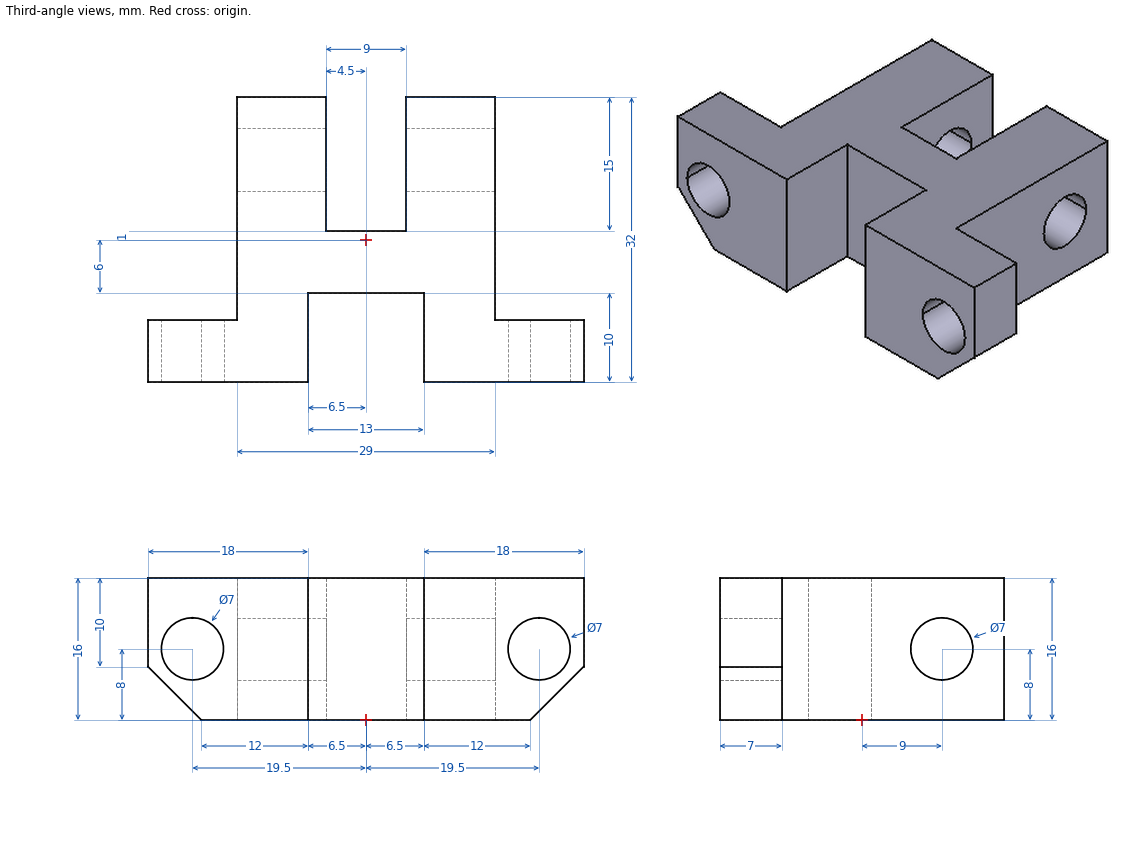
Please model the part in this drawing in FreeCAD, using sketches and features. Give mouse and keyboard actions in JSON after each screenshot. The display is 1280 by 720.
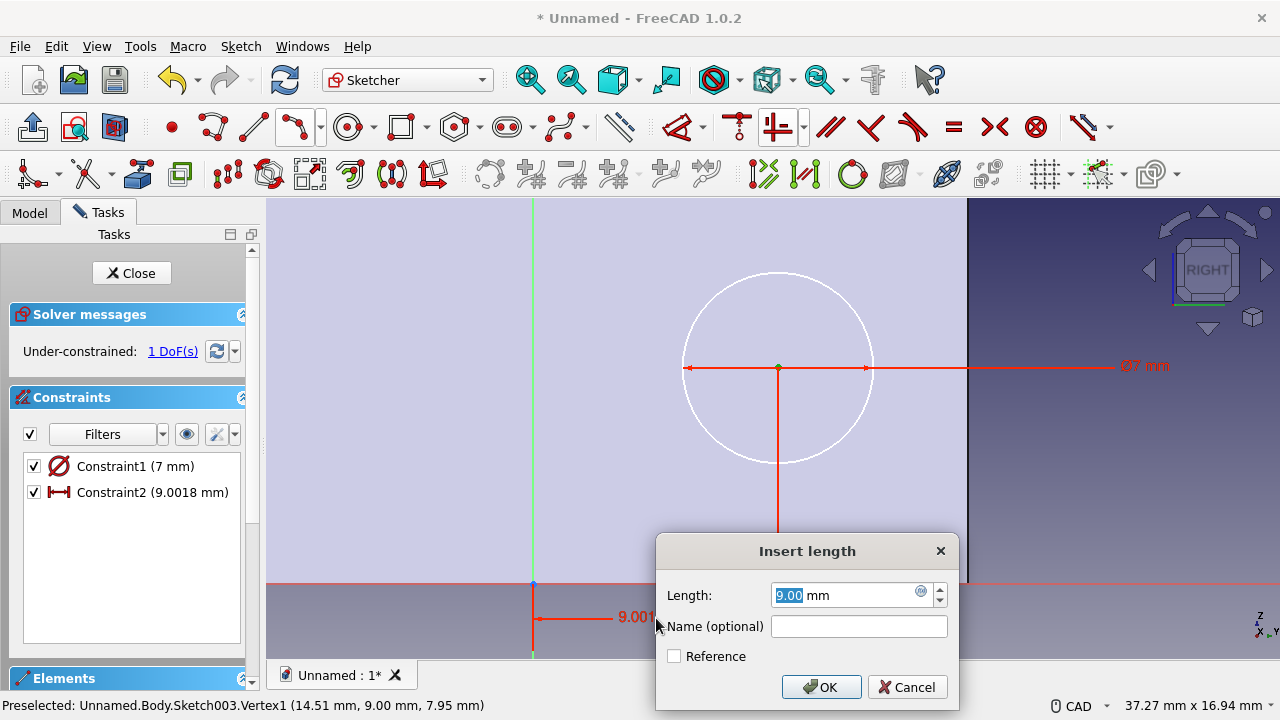
{"action": "type", "text": "9"}
{"action": "key", "text": "Return"}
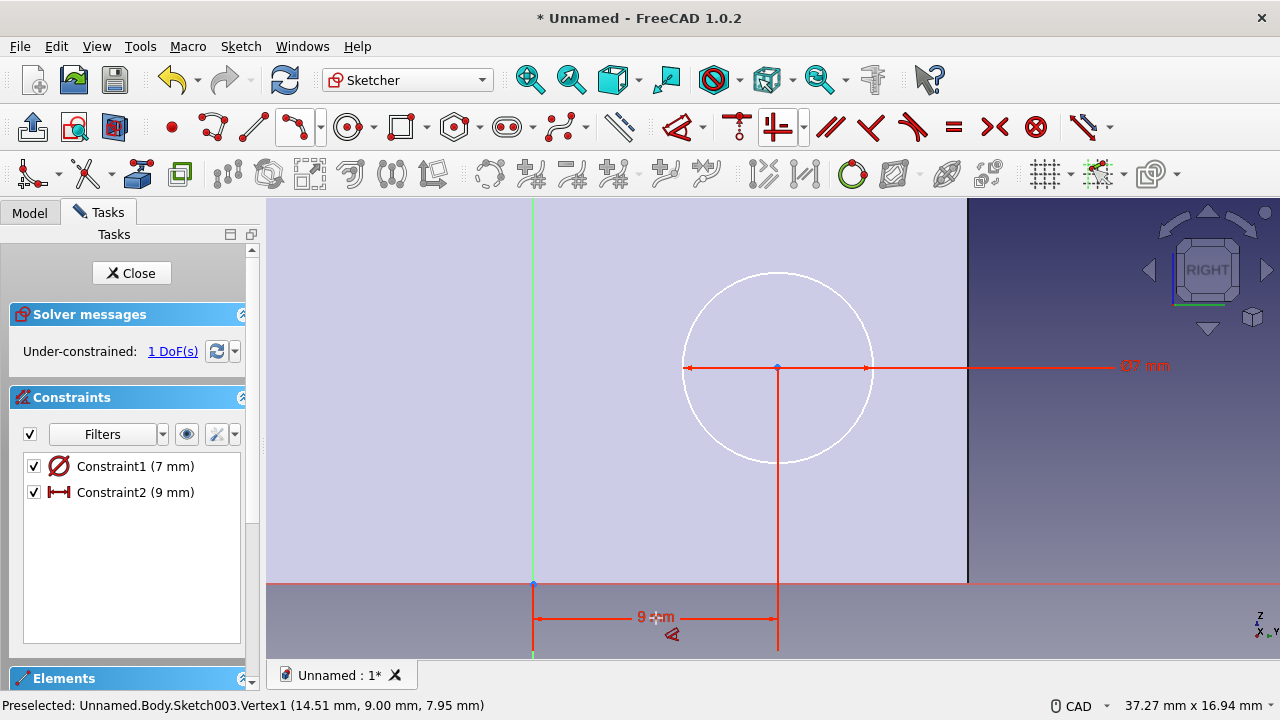
{"action": "left_click", "coordinate": [778, 368]}
{"action": "left_click", "coordinate": [499, 476]}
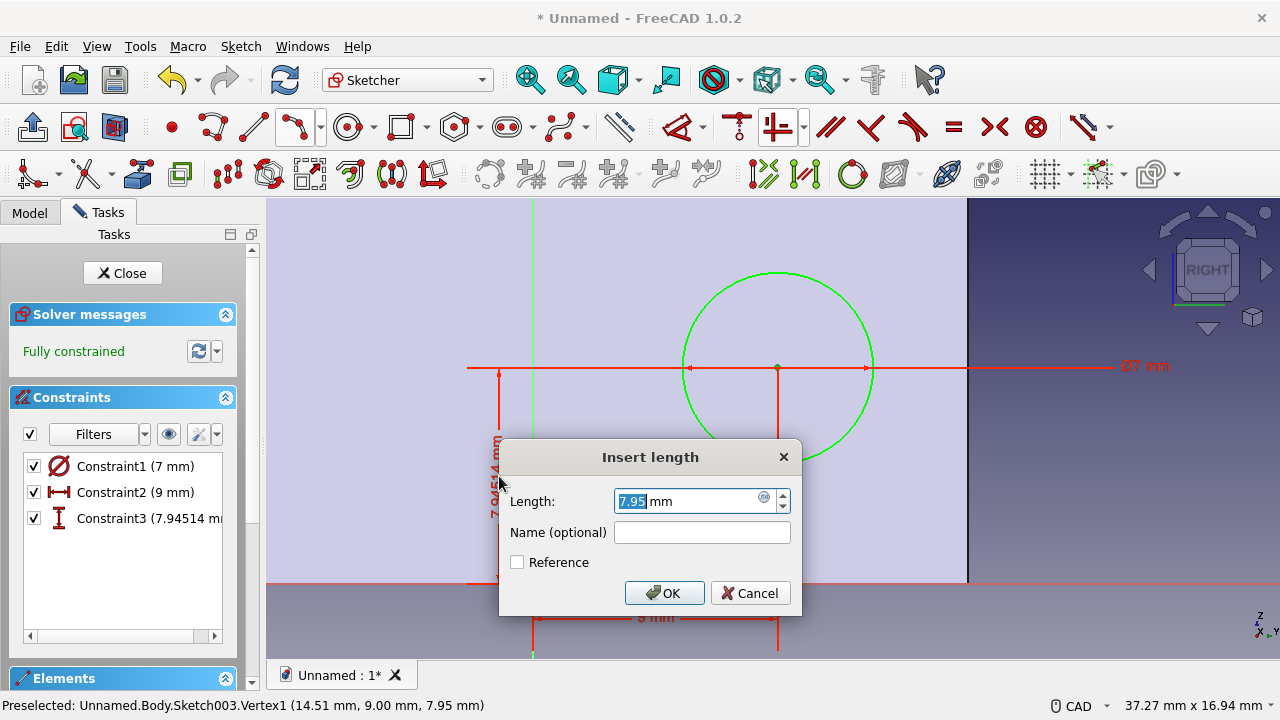
{"action": "type", "text": "8"}
{"action": "key", "text": "Return"}
{"action": "key", "text": "Escape"}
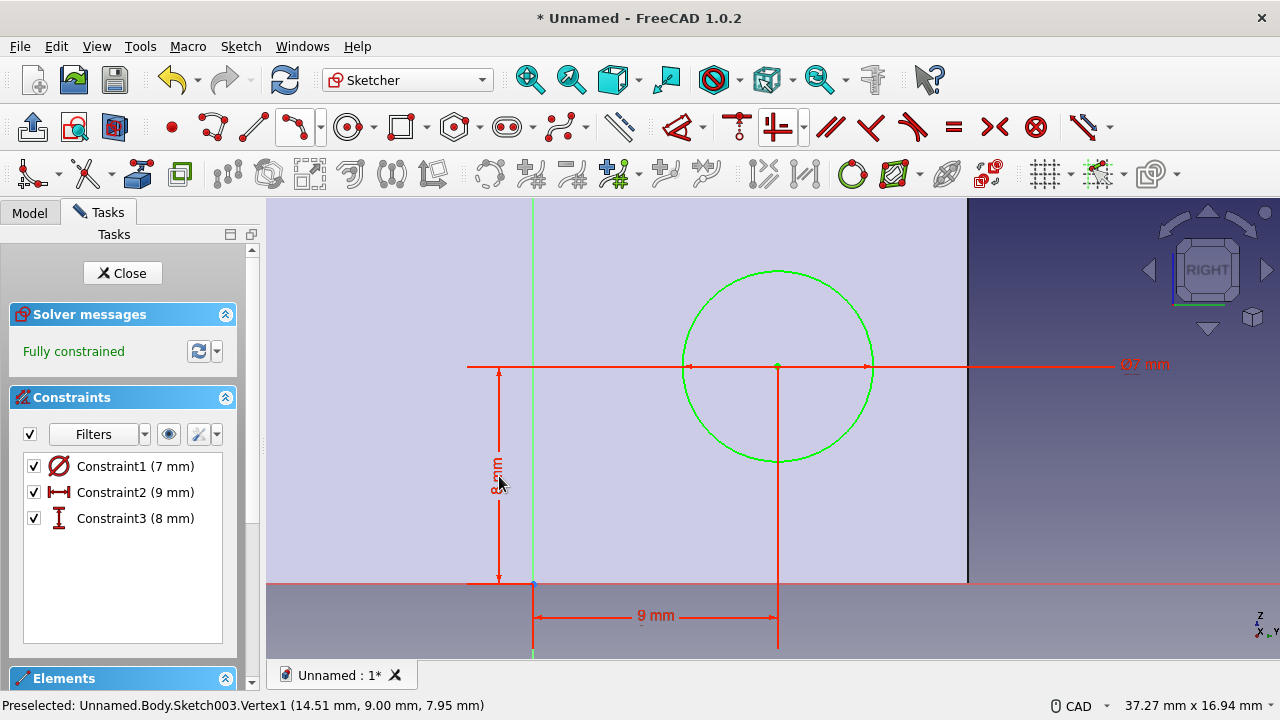
{"action": "left_click", "coordinate": [123, 273]}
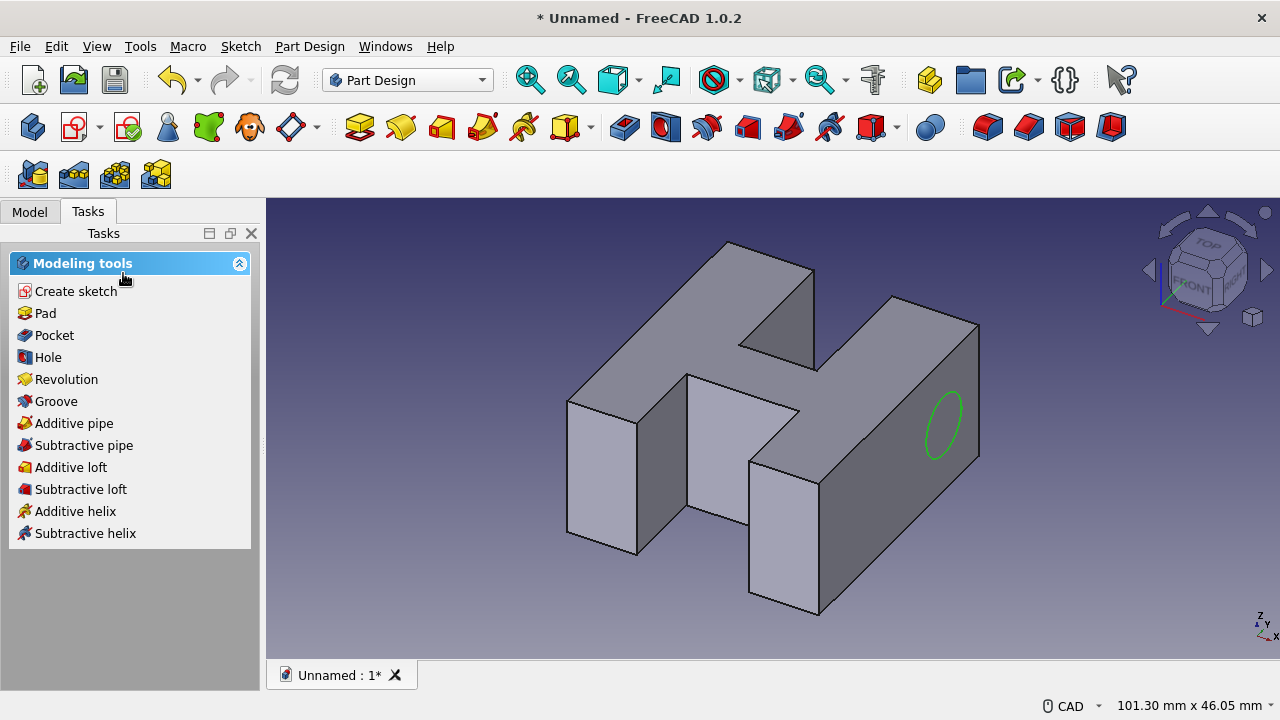
{"action": "left_click", "coordinate": [625, 128]}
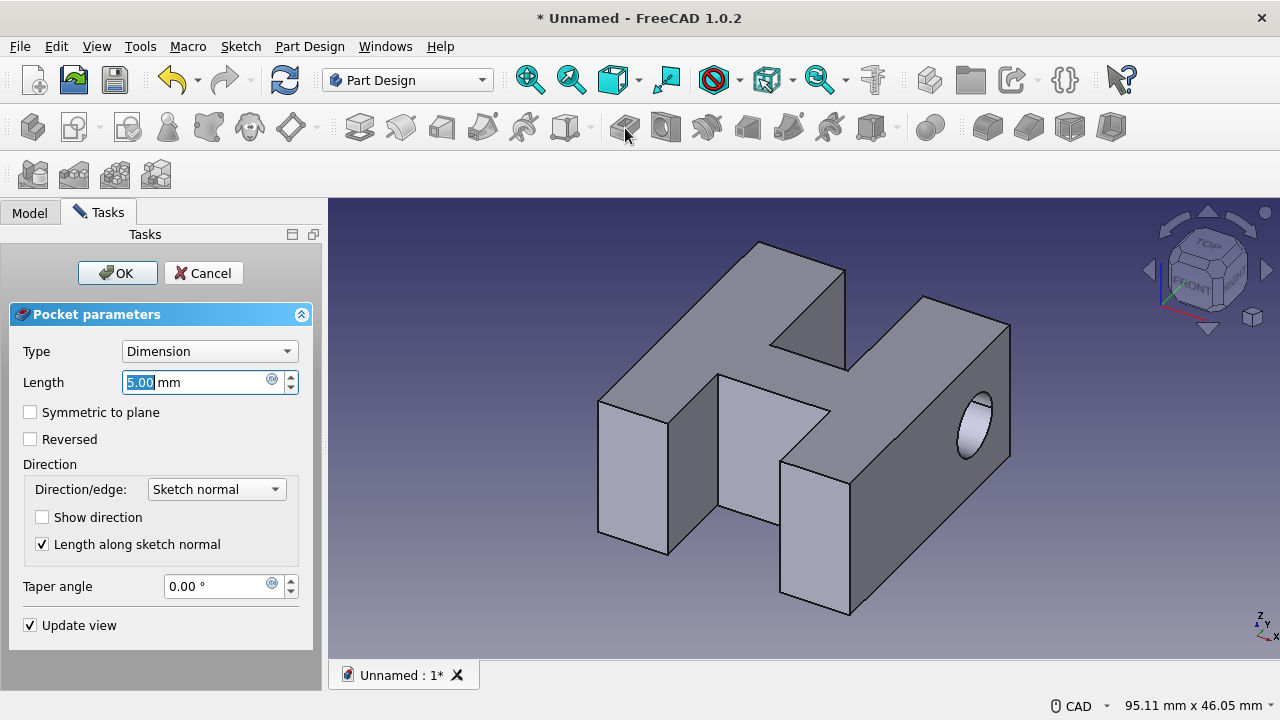
{"action": "left_click", "coordinate": [210, 352]}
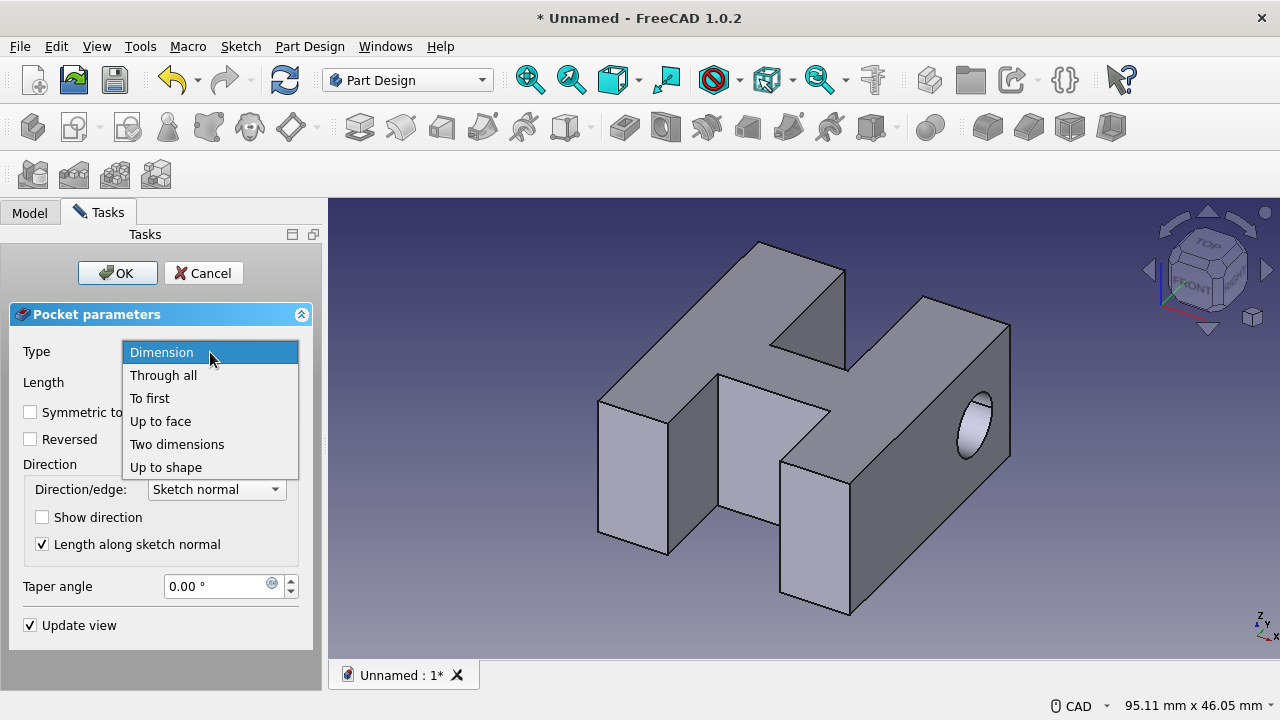
{"action": "left_click", "coordinate": [208, 376]}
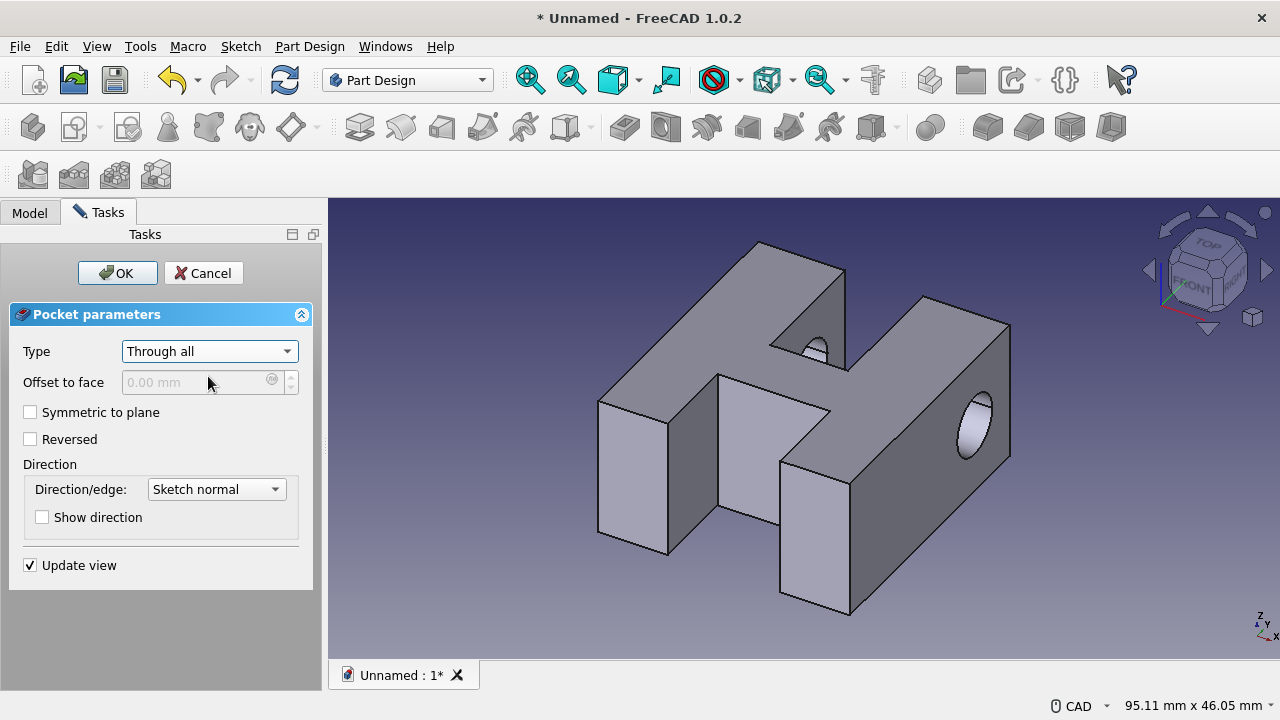
{"action": "left_click", "coordinate": [118, 273]}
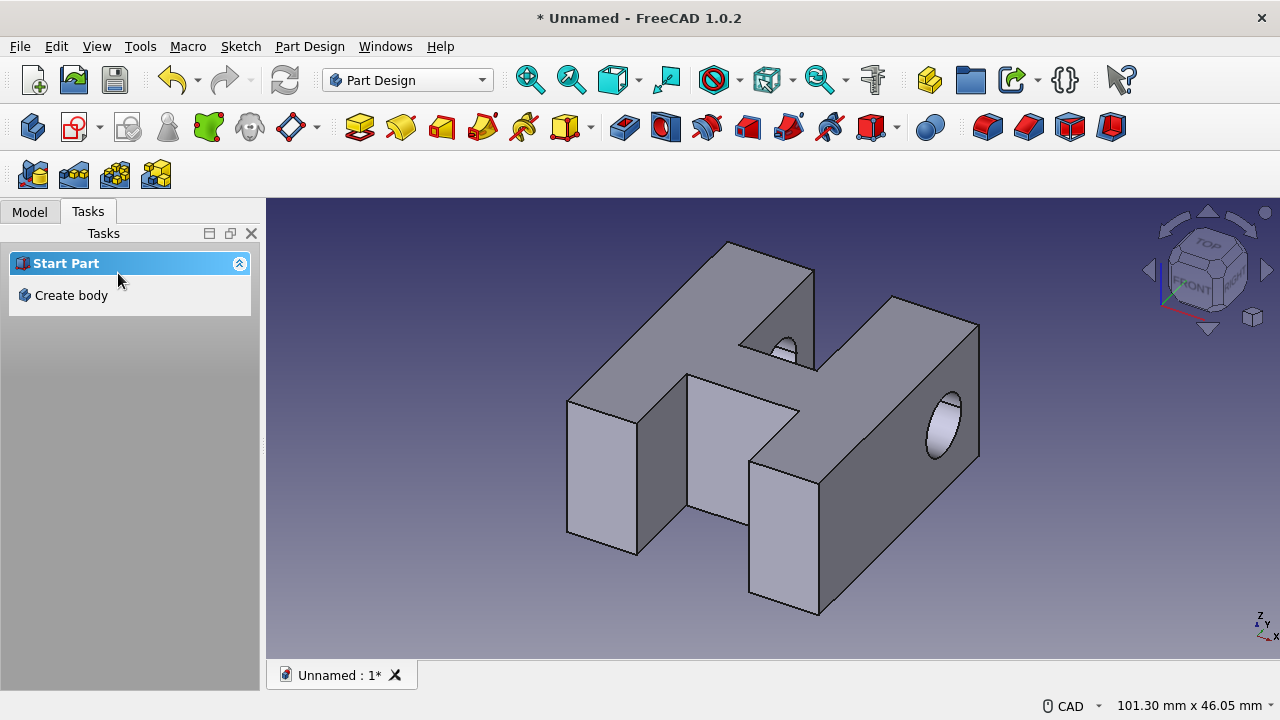
{"action": "left_click", "coordinate": [784, 518]}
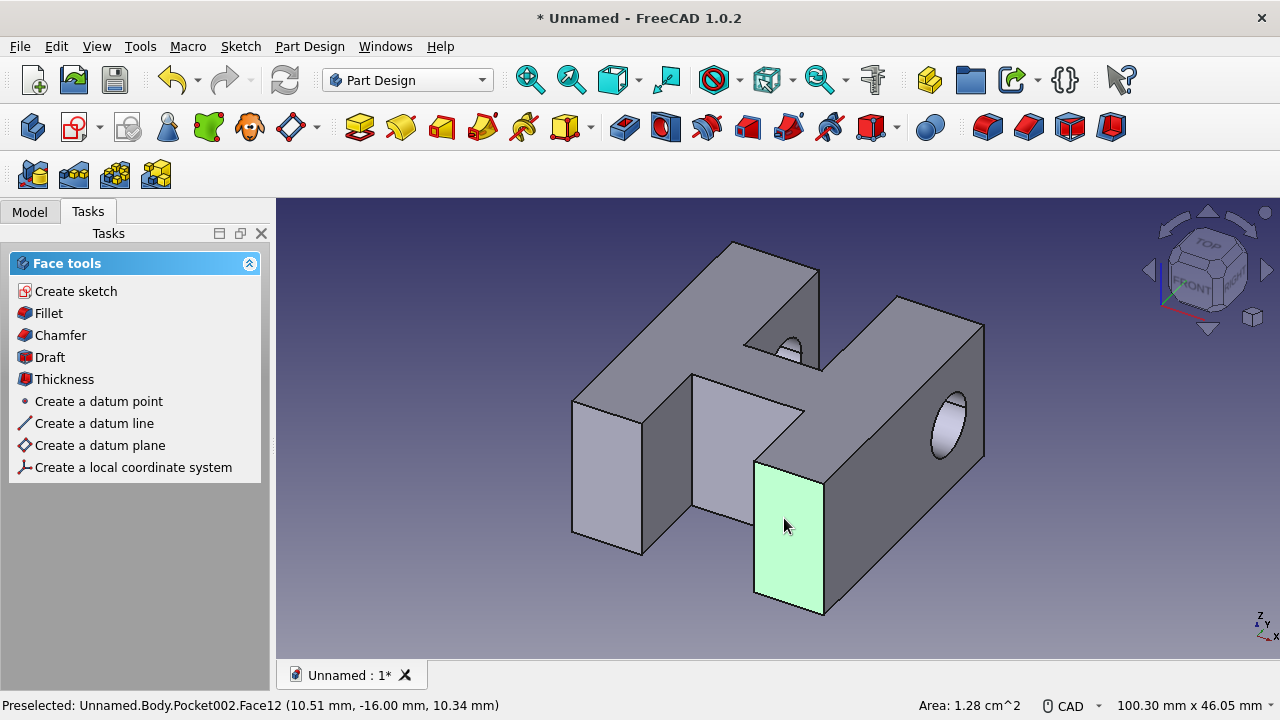
{"action": "left_click", "coordinate": [74, 128]}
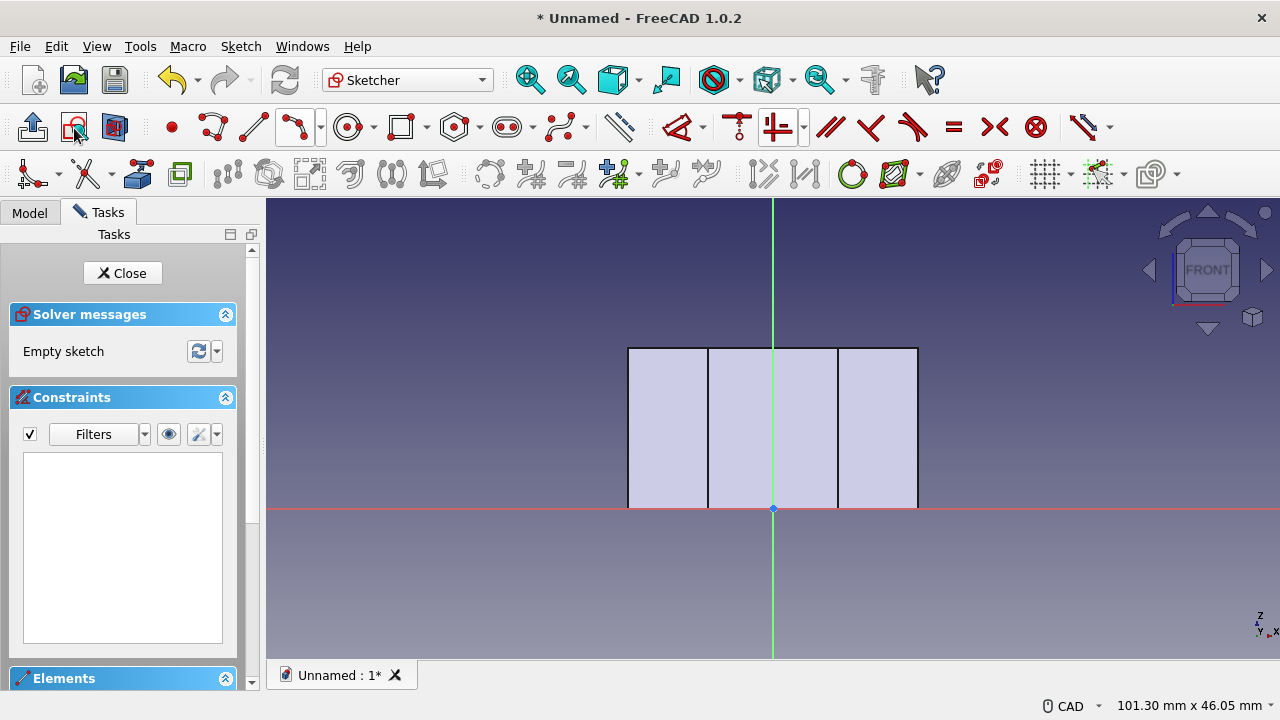
{"action": "scroll", "coordinate": [585, 429], "scroll_direction": "up", "scroll_amount": 3}